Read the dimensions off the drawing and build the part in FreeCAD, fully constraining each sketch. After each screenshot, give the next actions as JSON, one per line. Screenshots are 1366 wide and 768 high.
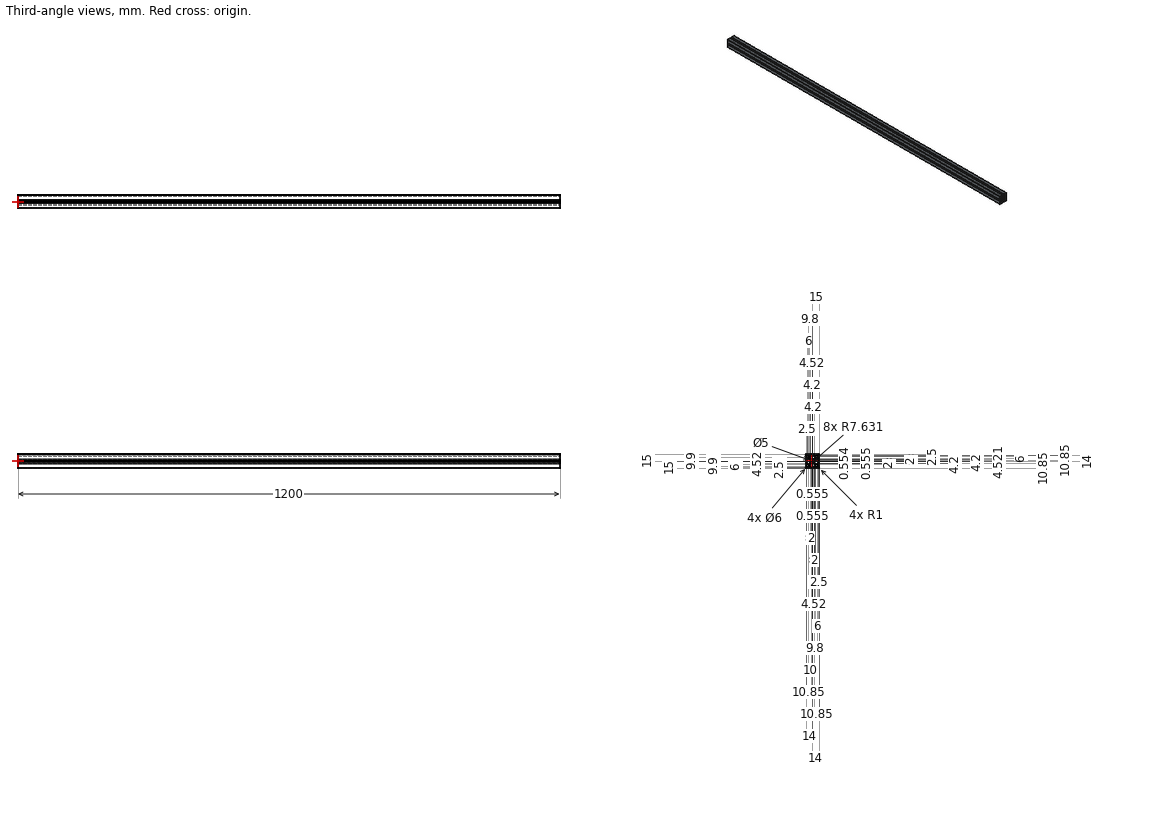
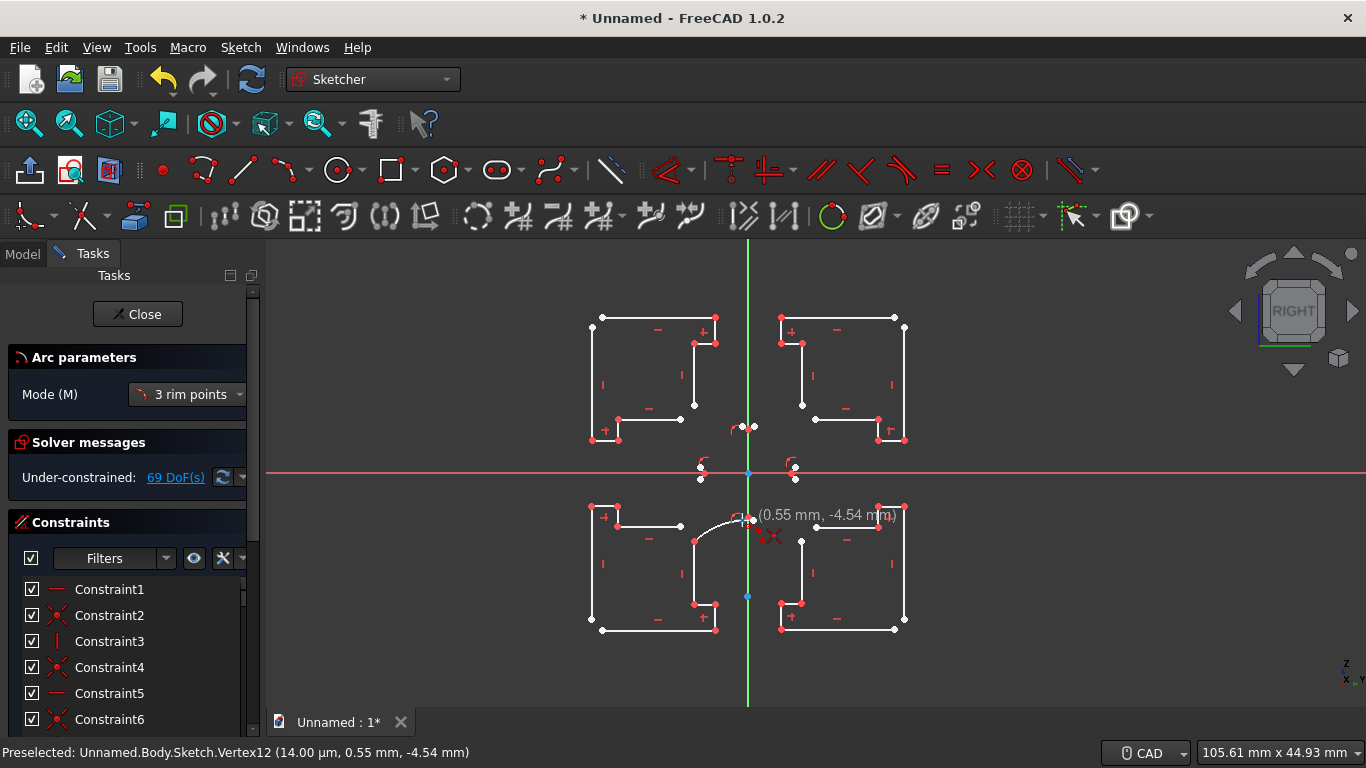
{"action": "left_click", "coordinate": [802, 541]}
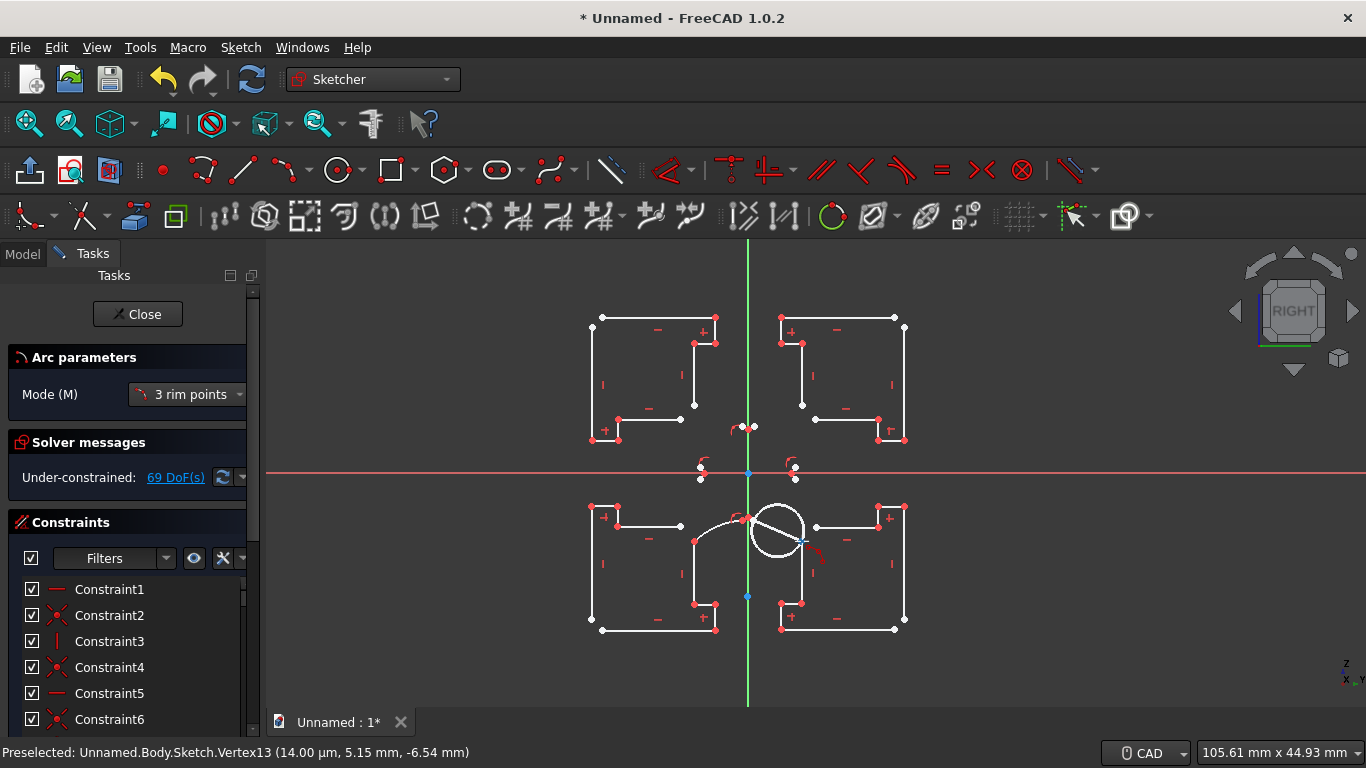
{"action": "scroll", "coordinate": [780, 526], "scroll_direction": "up", "scroll_amount": 7}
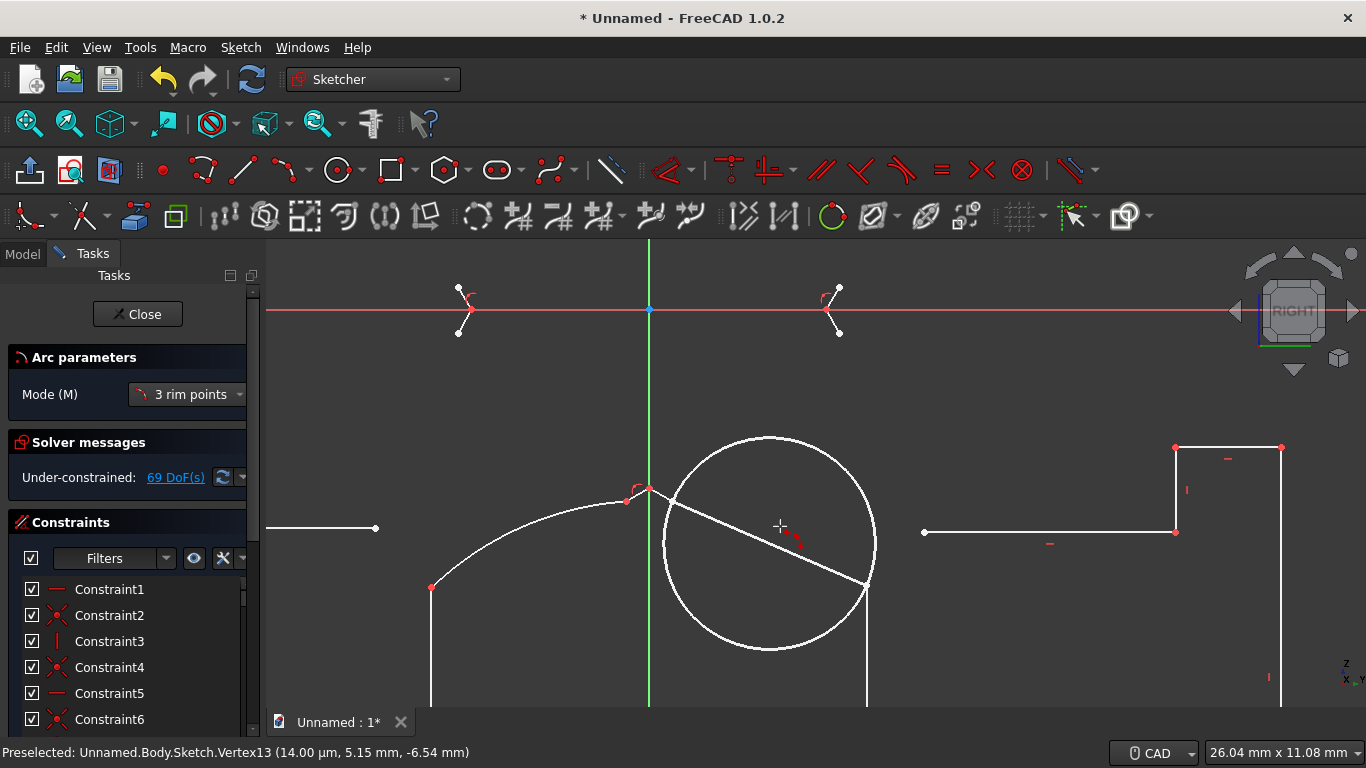
{"action": "left_click", "coordinate": [777, 526]}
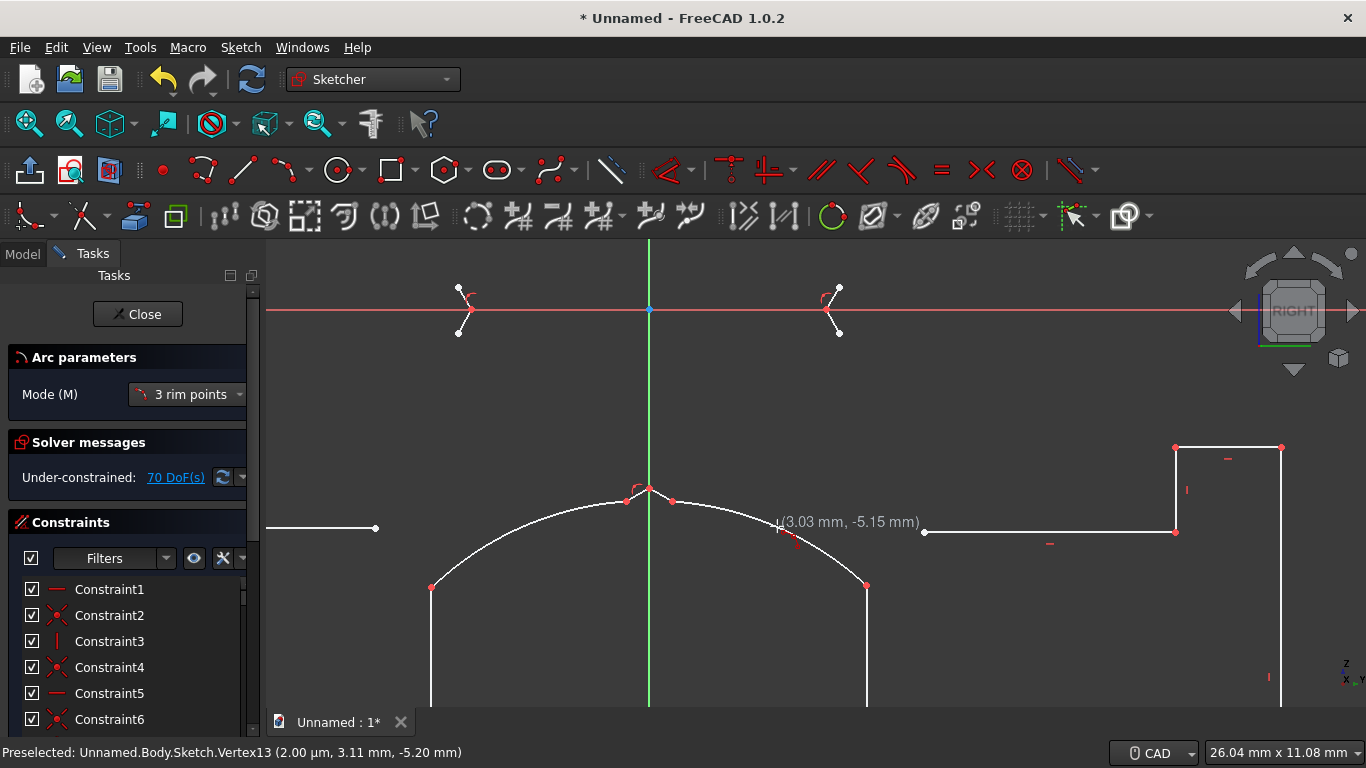
{"action": "scroll", "coordinate": [780, 527], "scroll_direction": "down", "scroll_amount": 7}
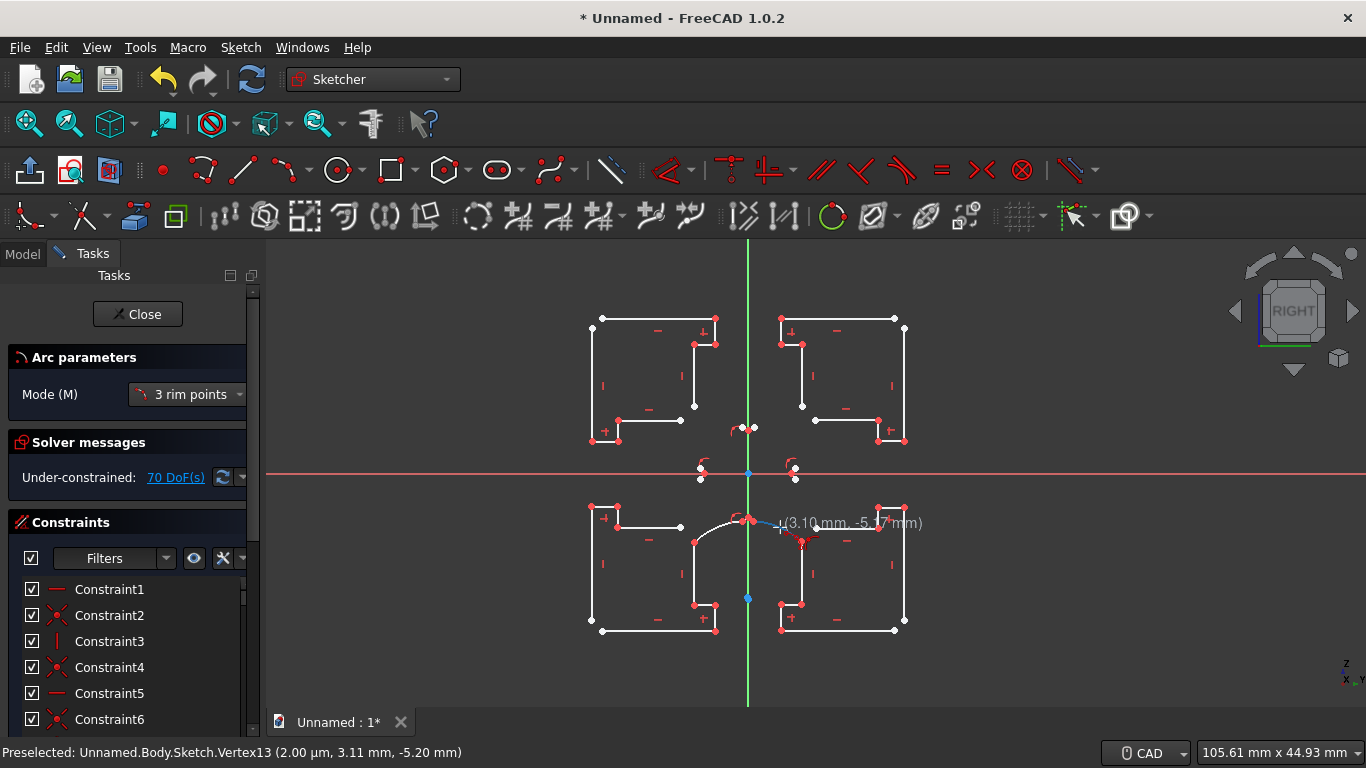
{"action": "left_click", "coordinate": [894, 631]}
{"action": "left_click", "coordinate": [904, 621]}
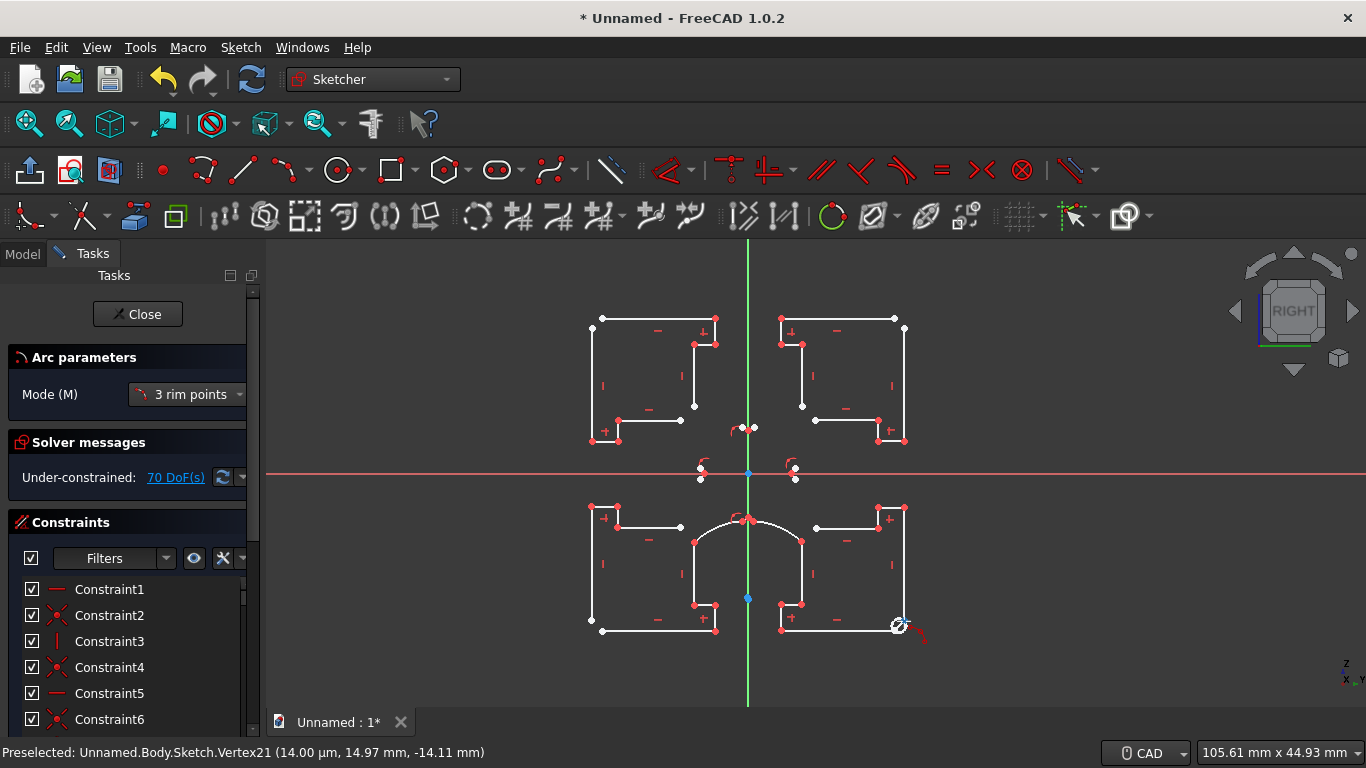
{"action": "scroll", "coordinate": [901, 627], "scroll_direction": "up", "scroll_amount": 9}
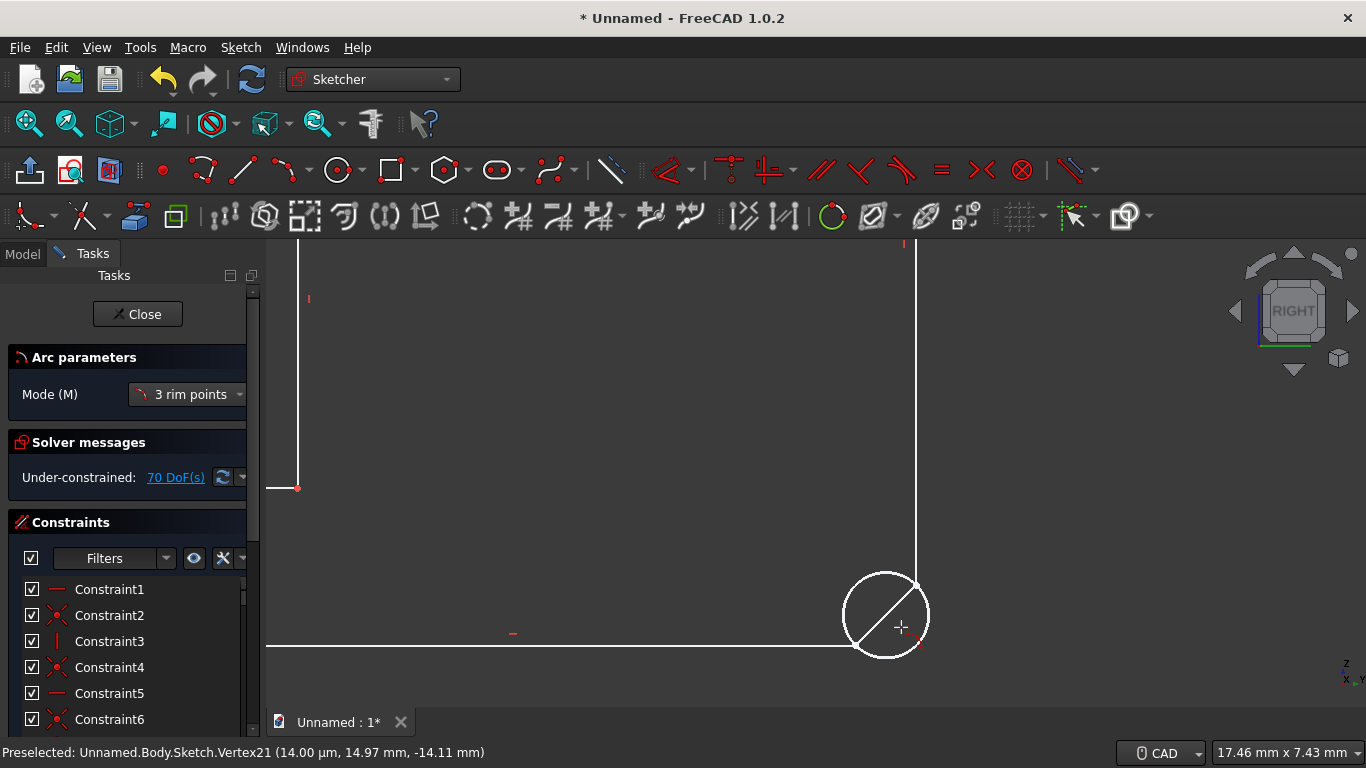
{"action": "left_click", "coordinate": [900, 623]}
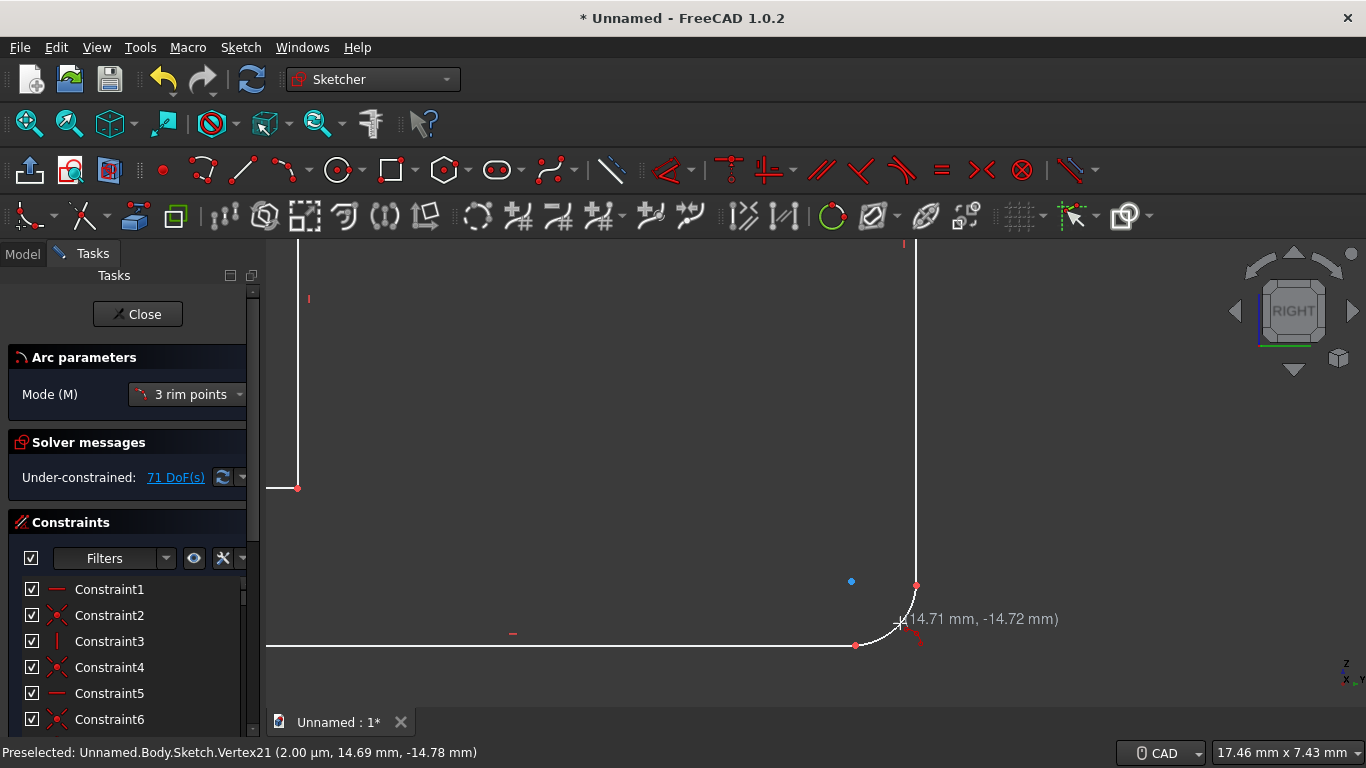
{"action": "scroll", "coordinate": [901, 627], "scroll_direction": "down", "scroll_amount": 9}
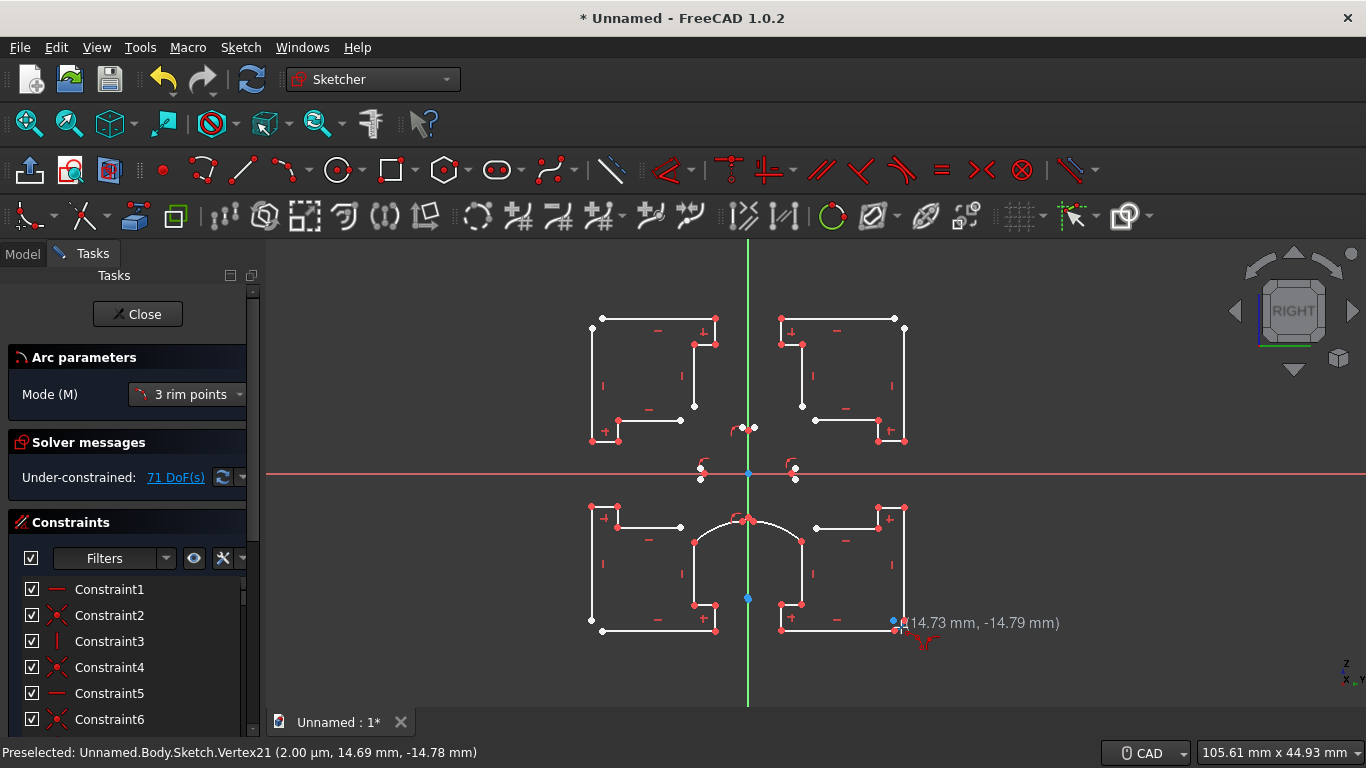
{"action": "left_click", "coordinate": [816, 529]}